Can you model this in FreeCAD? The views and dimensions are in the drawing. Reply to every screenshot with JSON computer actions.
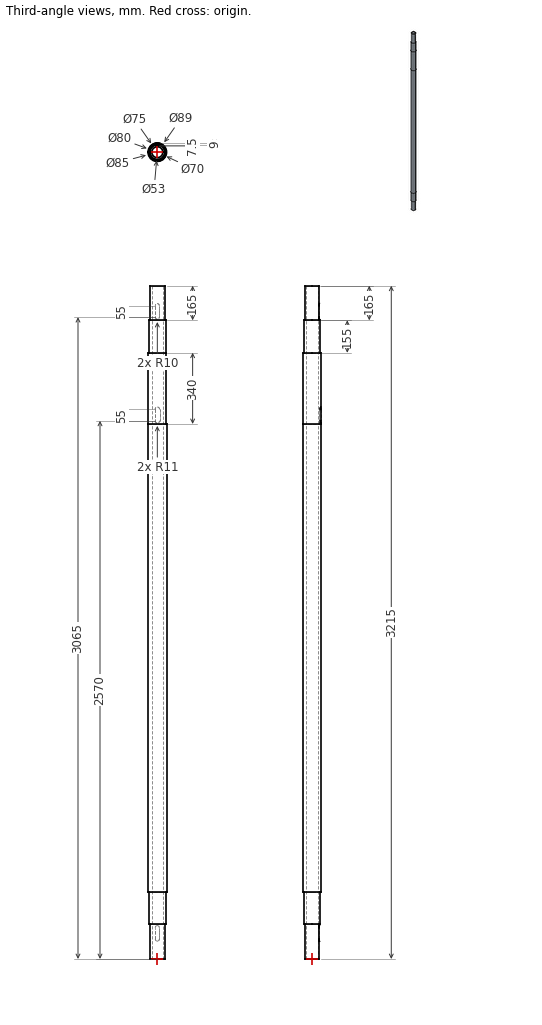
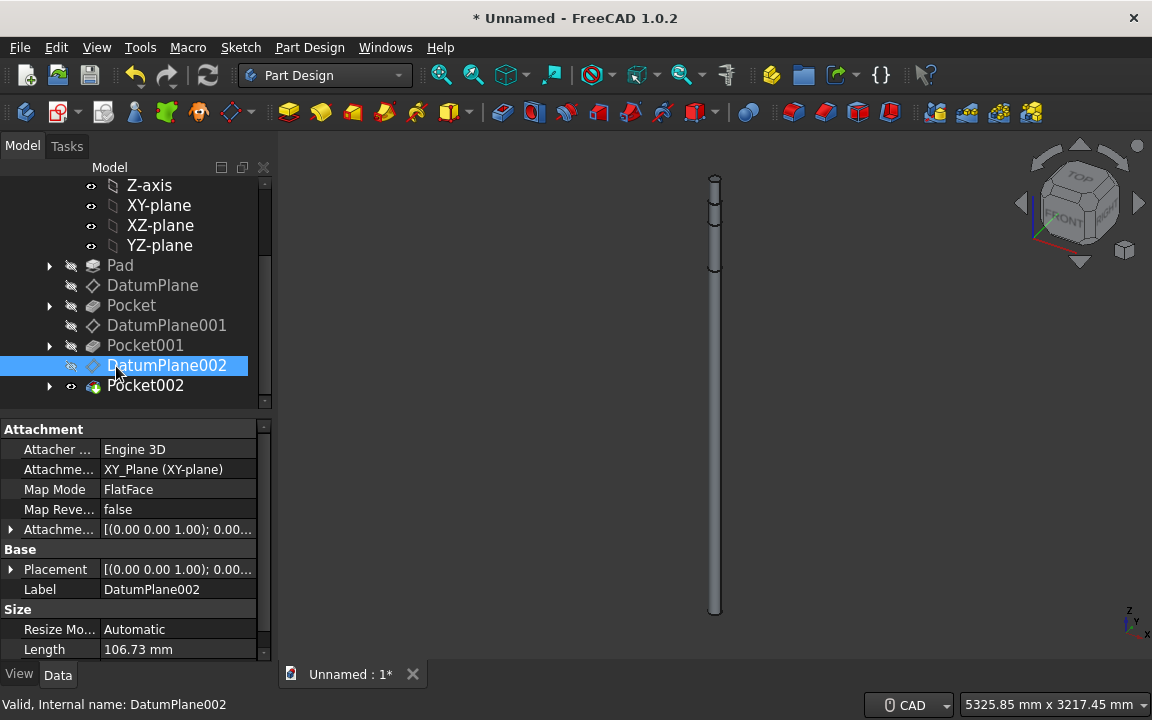
{"action": "scroll", "coordinate": [715, 178], "scroll_direction": "up", "scroll_amount": 4}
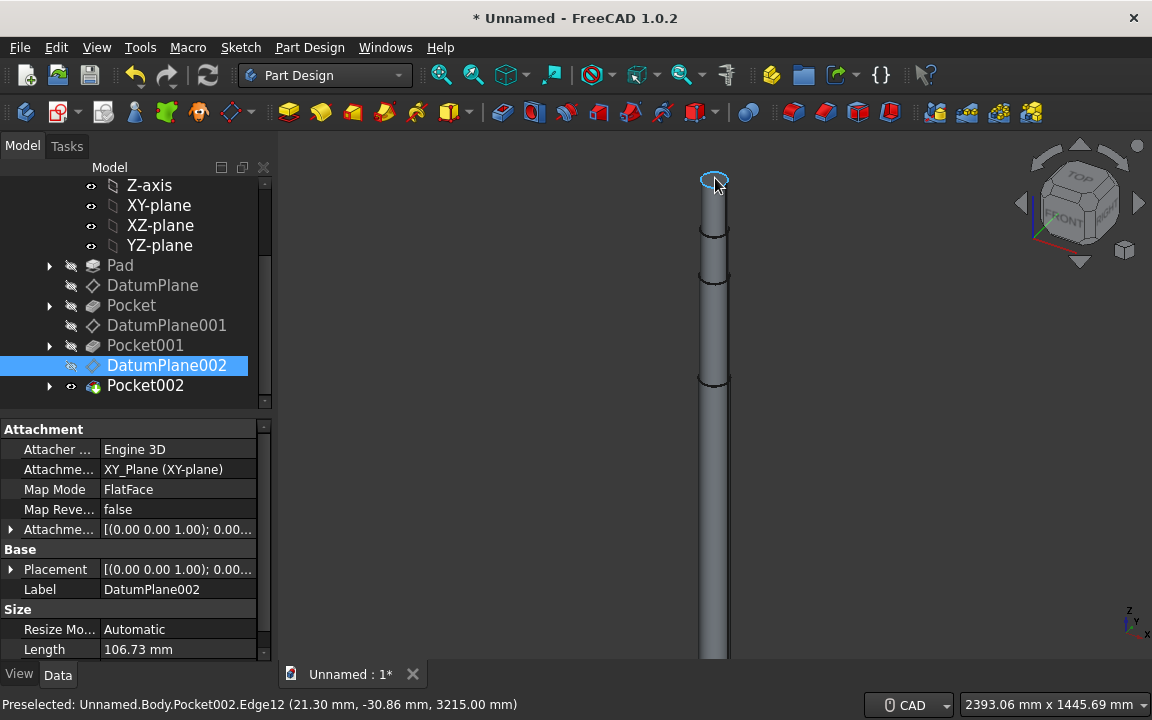
{"action": "left_click", "coordinate": [716, 177]}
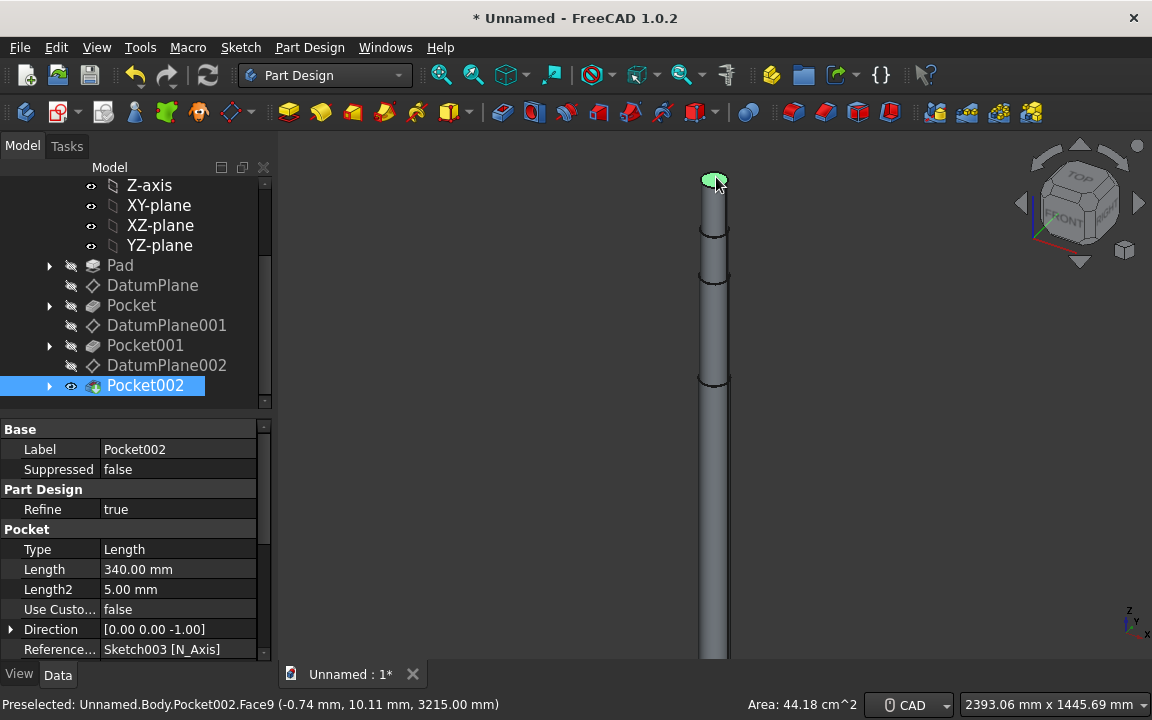
{"action": "left_click", "coordinate": [58, 112]}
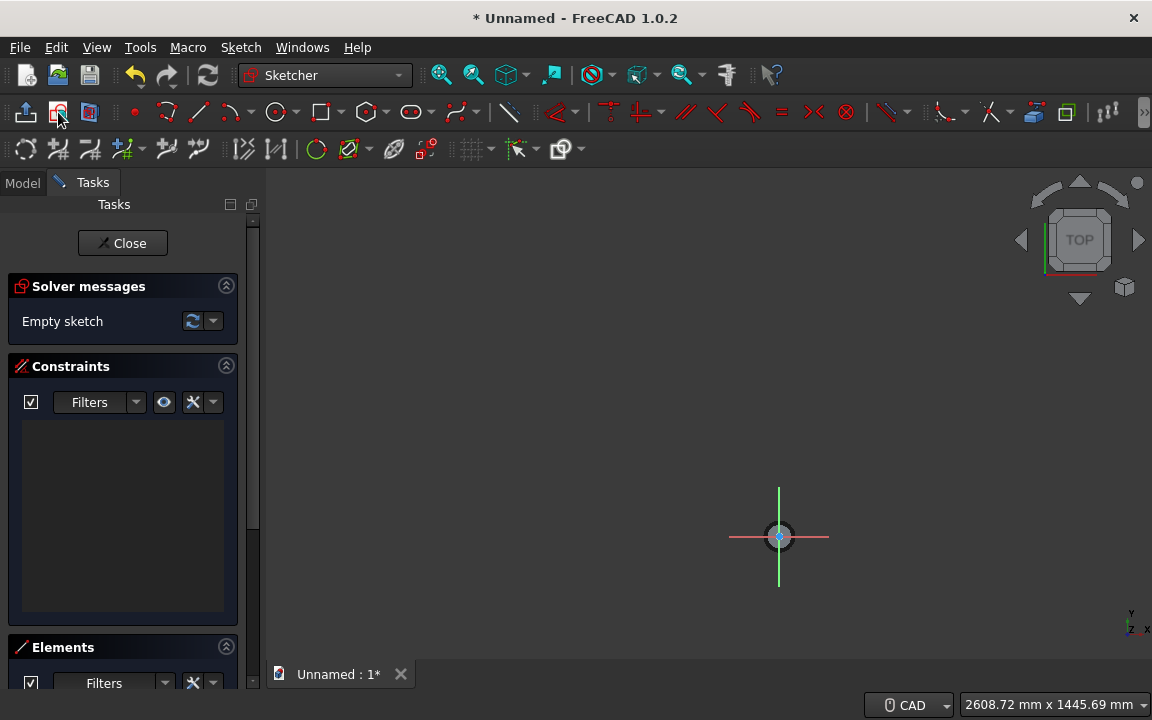
{"action": "scroll", "coordinate": [788, 545], "scroll_direction": "up", "scroll_amount": 14}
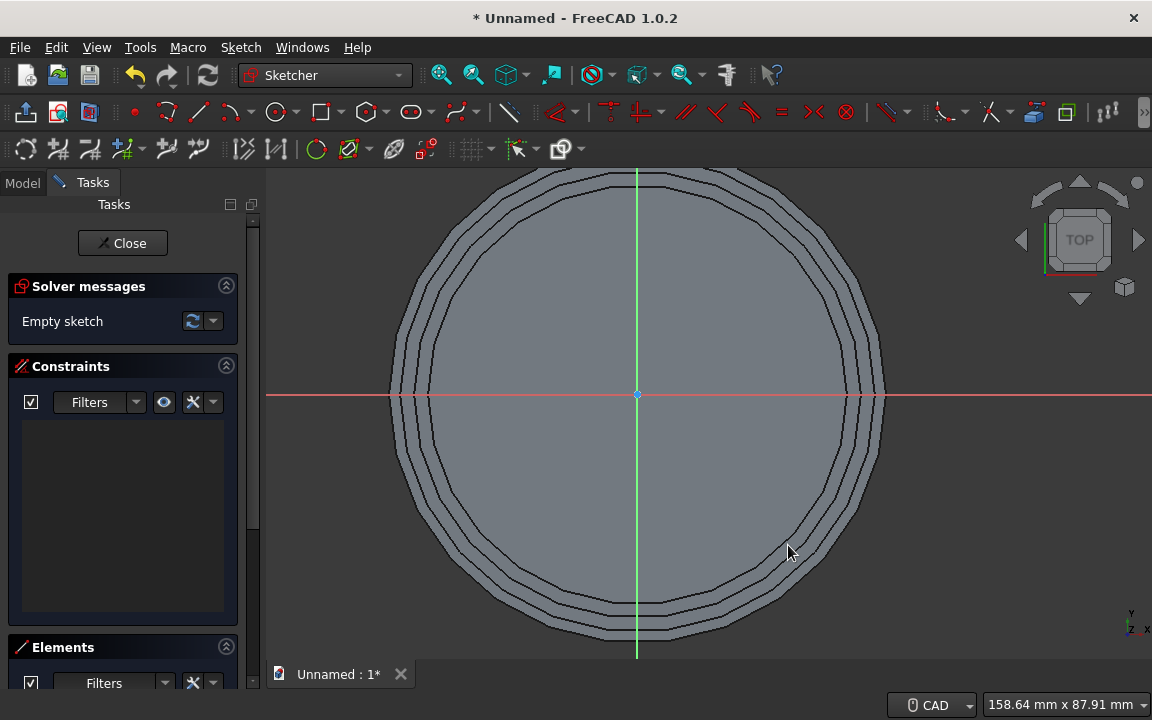
{"action": "left_click", "coordinate": [276, 112]}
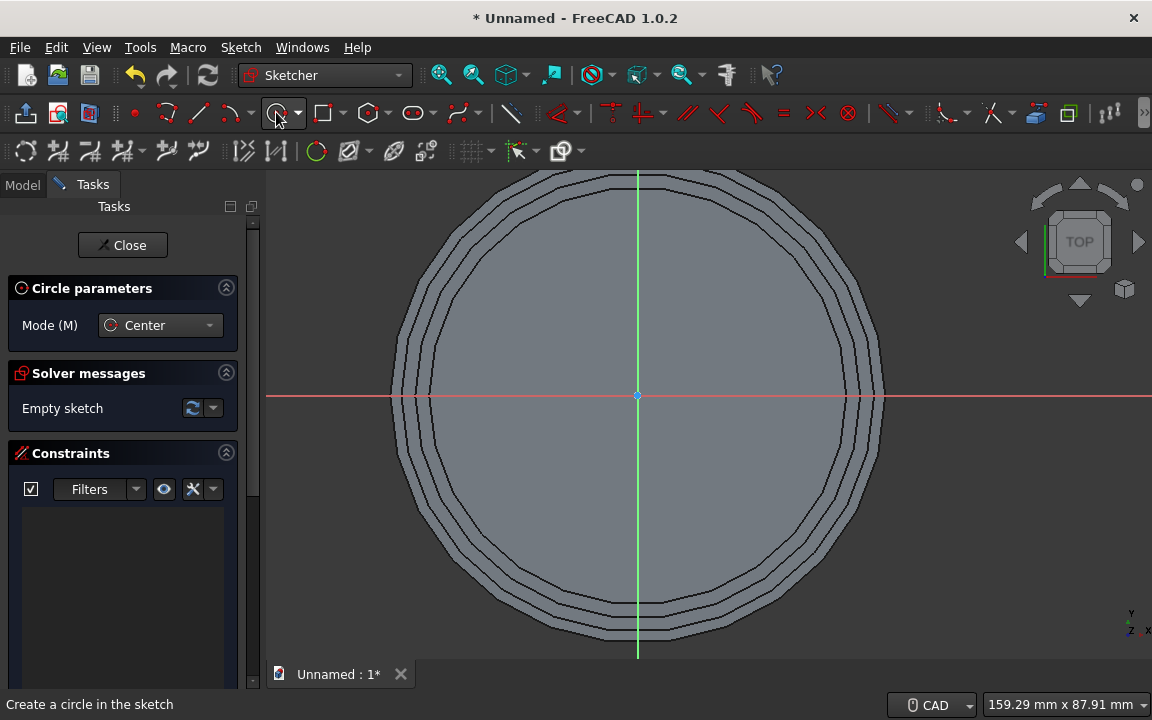
{"action": "left_click", "coordinate": [638, 396]}
{"action": "mouse_move", "coordinate": [742, 291]}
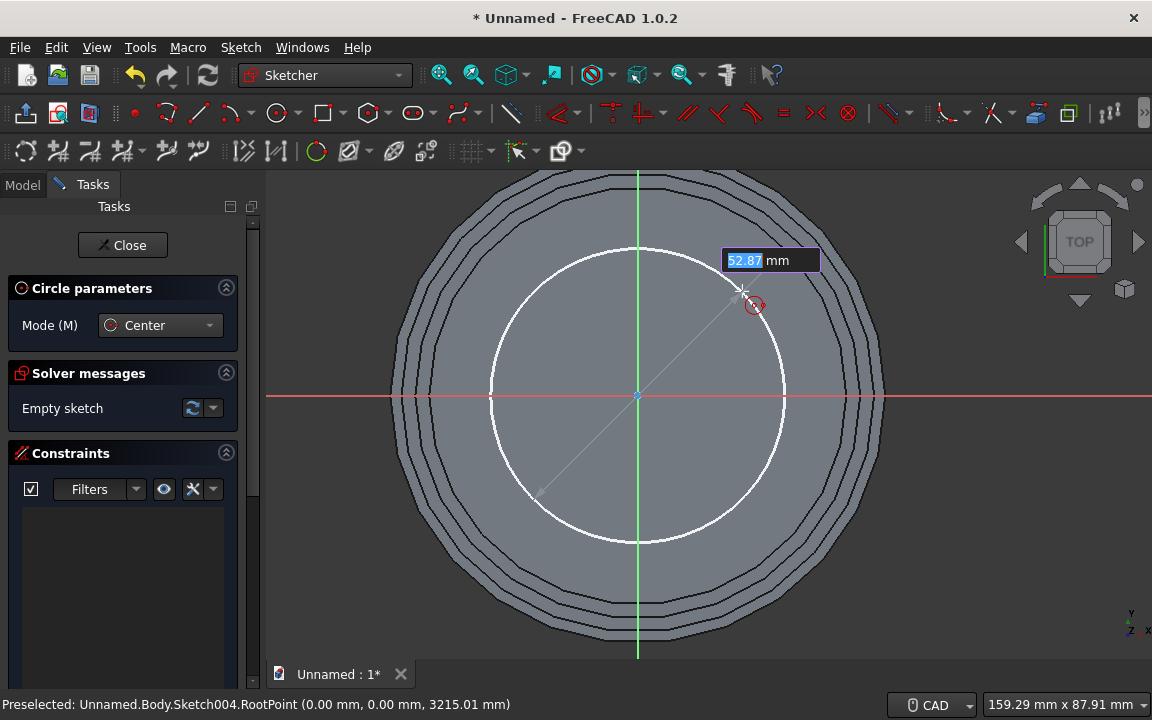
{"action": "type", "text": "53"}
{"action": "key", "text": "Return"}
{"action": "key", "text": "Escape"}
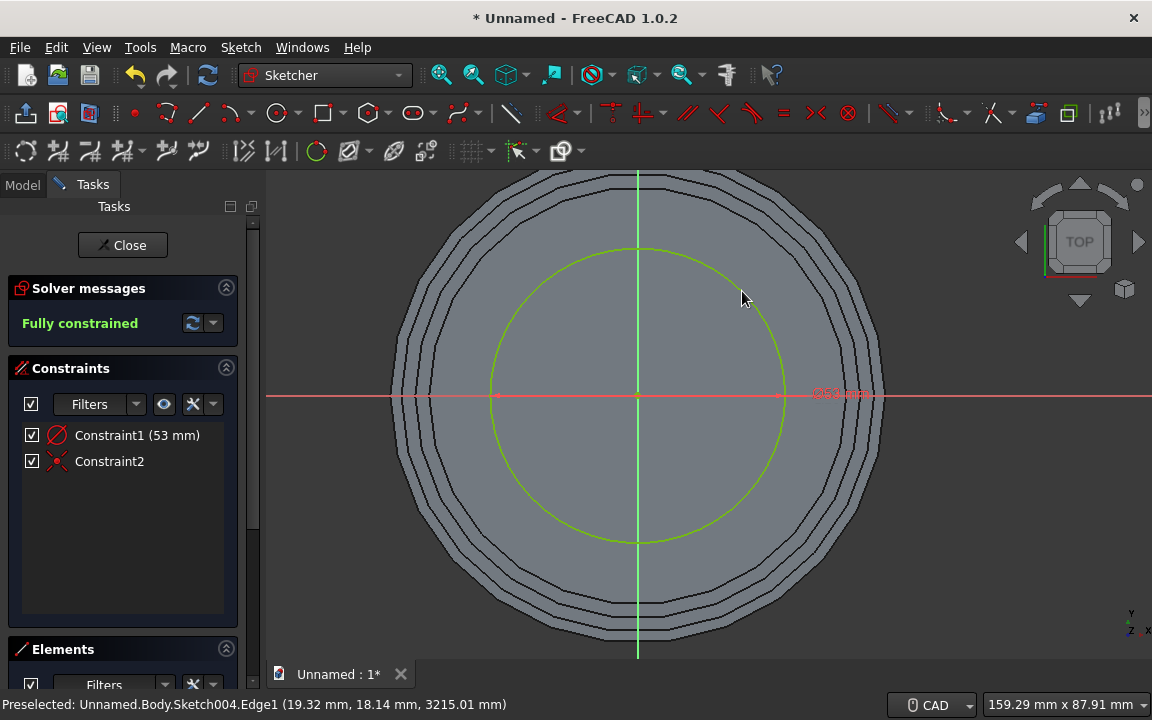
{"action": "left_click", "coordinate": [123, 245]}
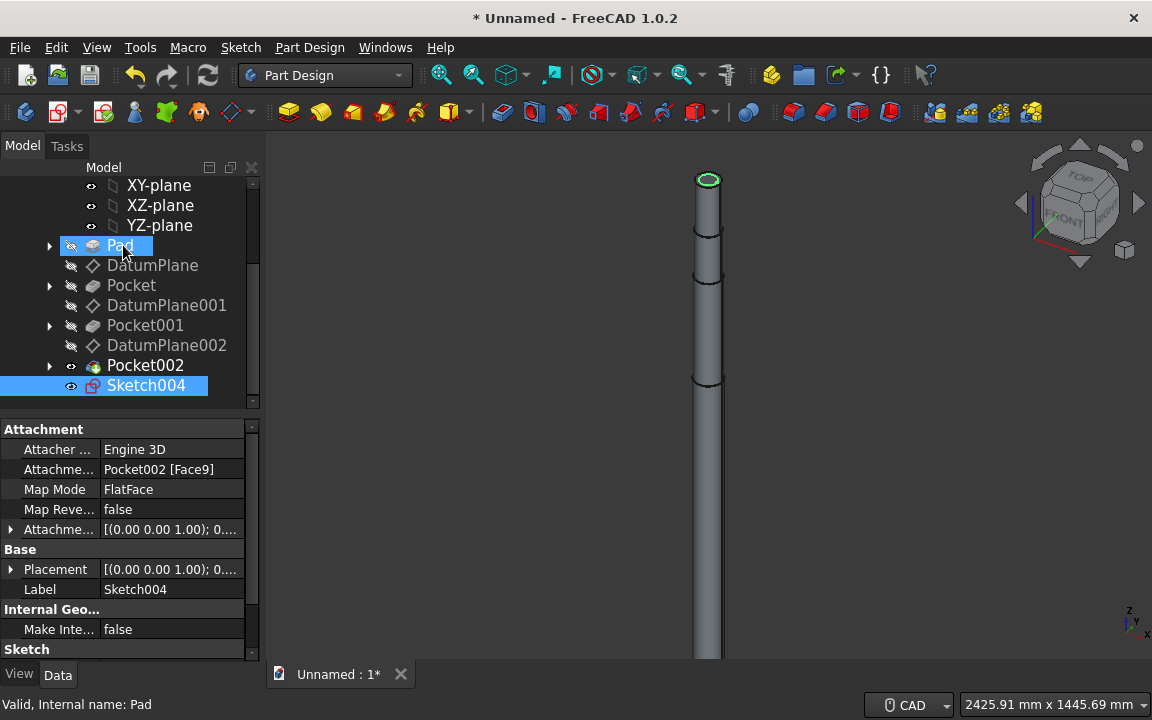
{"action": "left_click", "coordinate": [504, 112]}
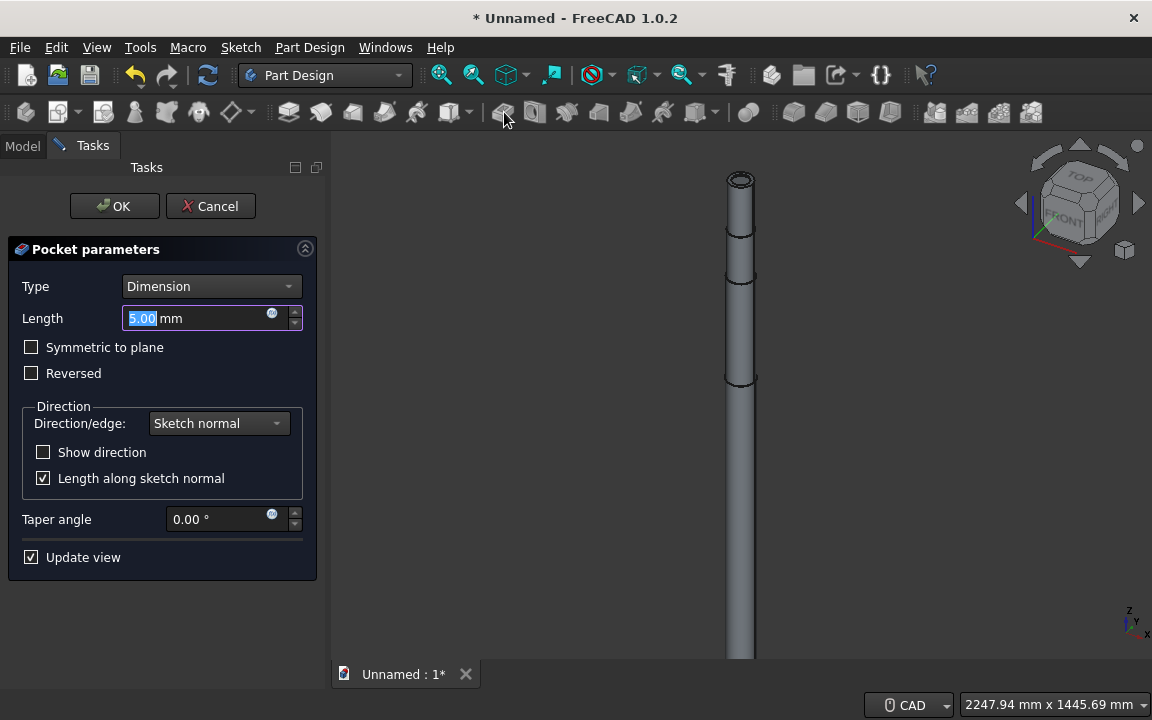
{"action": "left_click", "coordinate": [212, 286]}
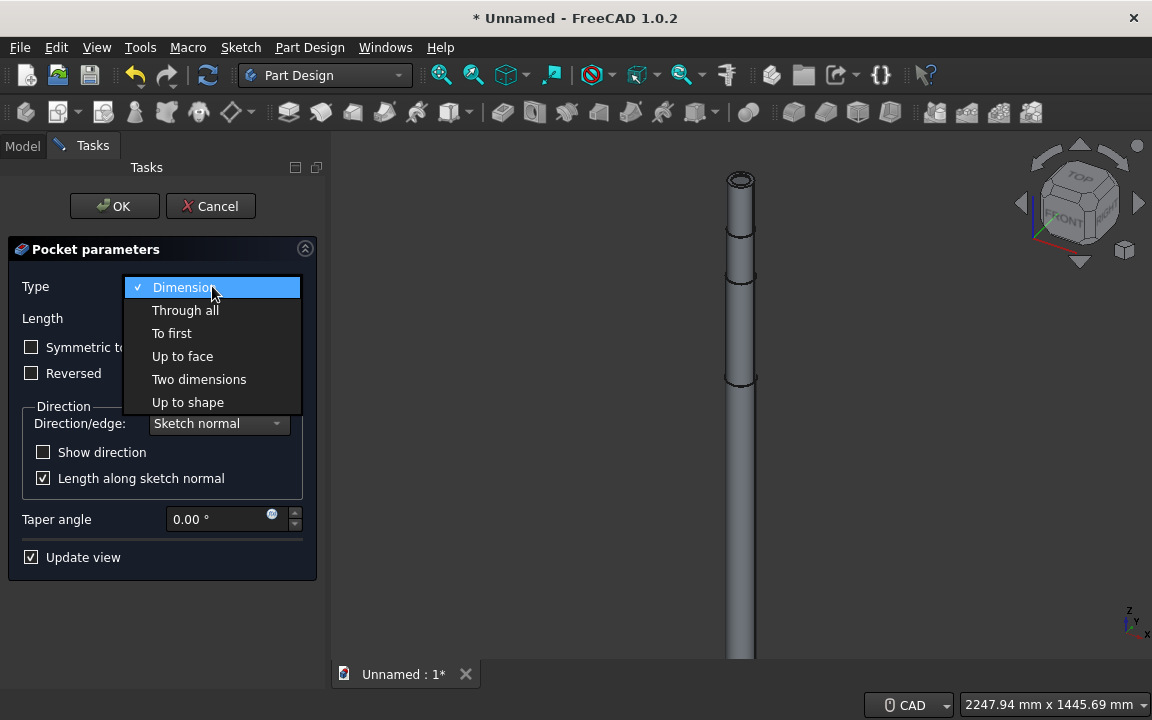
{"action": "left_click", "coordinate": [212, 310]}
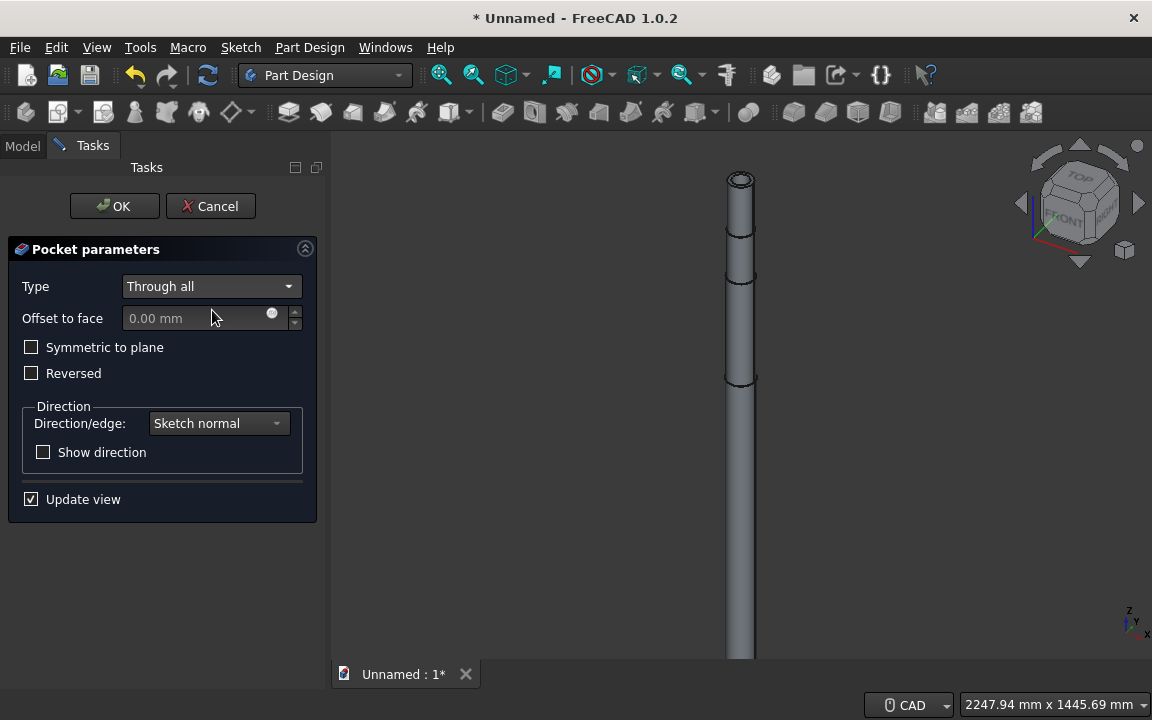
{"action": "left_click", "coordinate": [115, 206]}